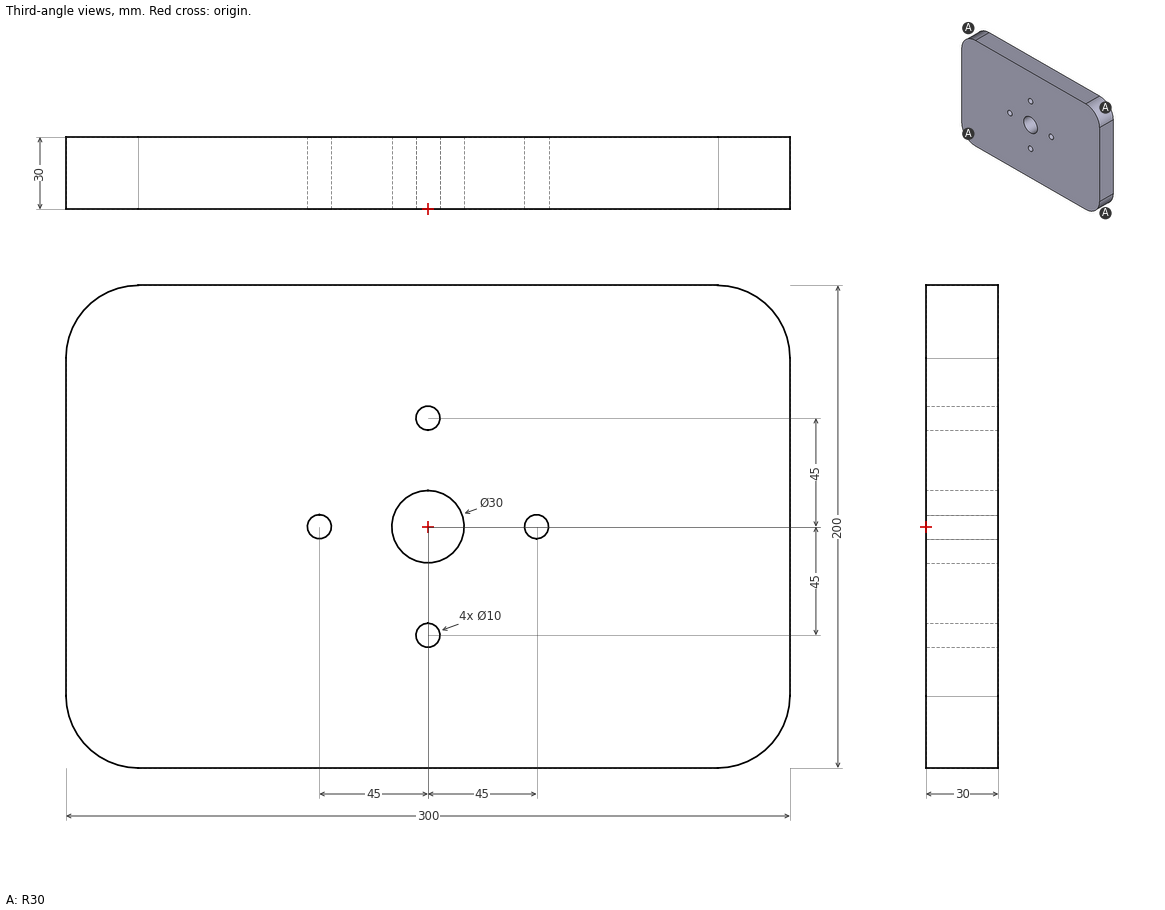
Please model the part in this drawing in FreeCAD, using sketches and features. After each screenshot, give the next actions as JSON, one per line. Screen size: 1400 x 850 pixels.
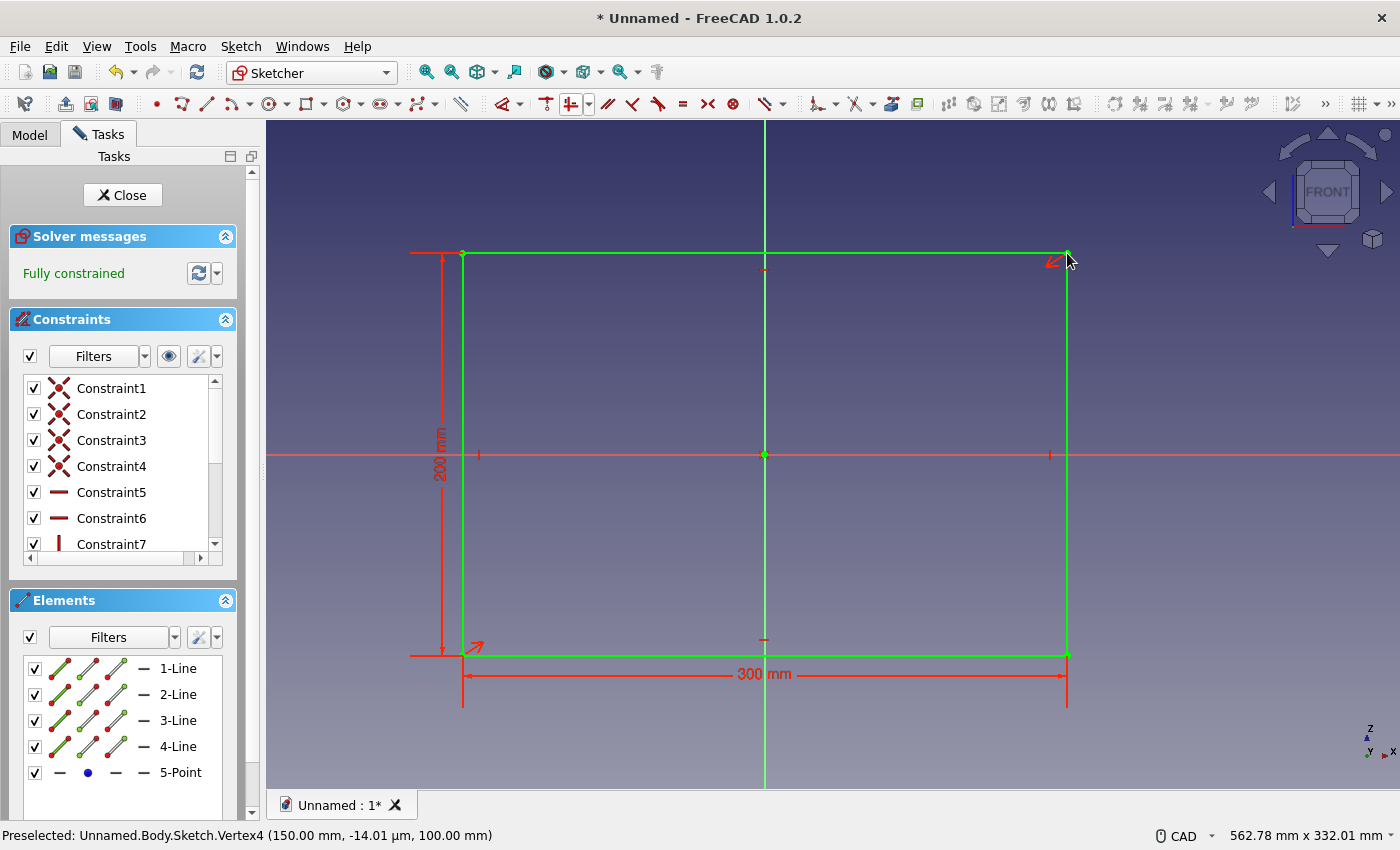
{"action": "left_click", "coordinate": [123, 195]}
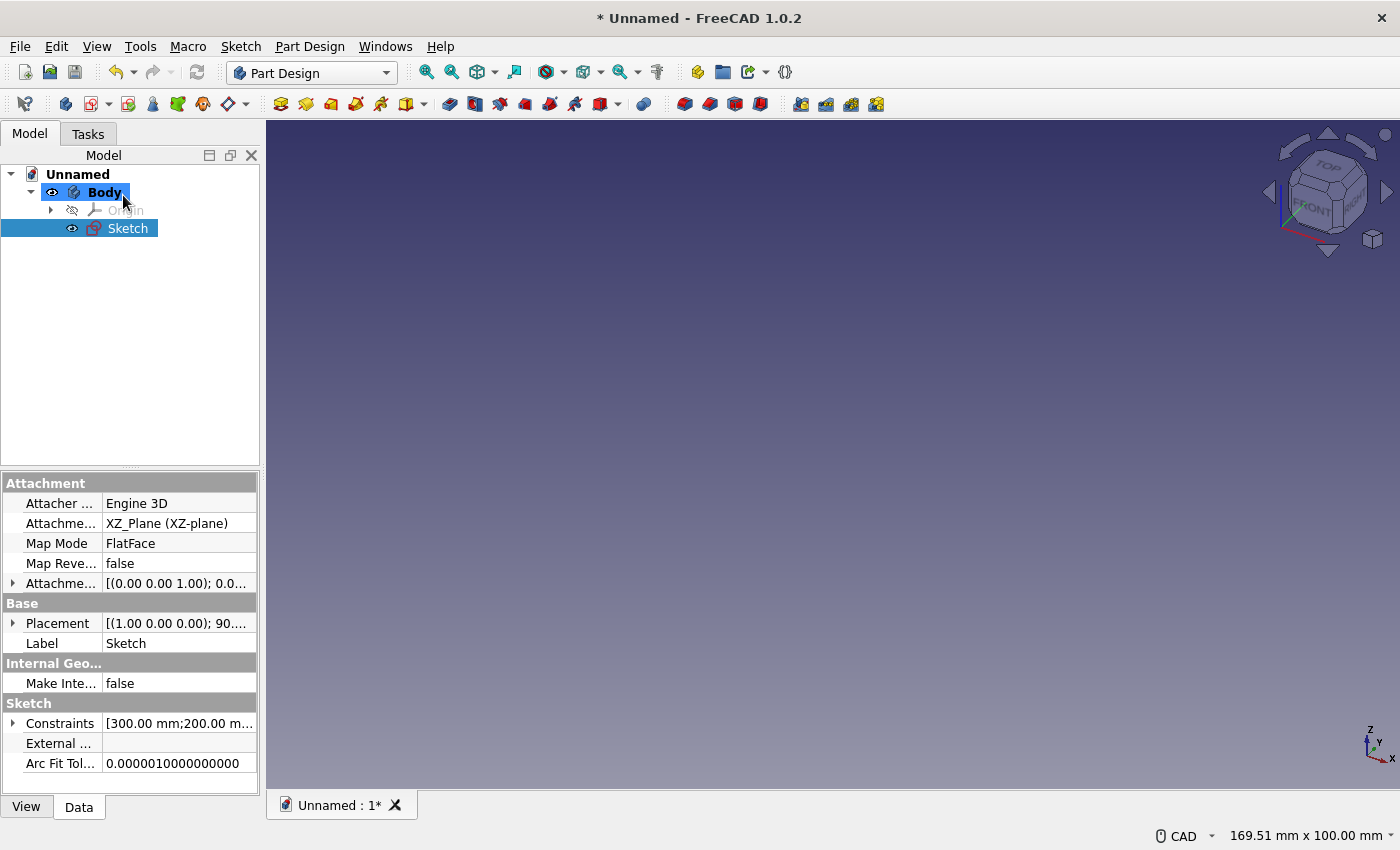
{"action": "left_click", "coordinate": [281, 104]}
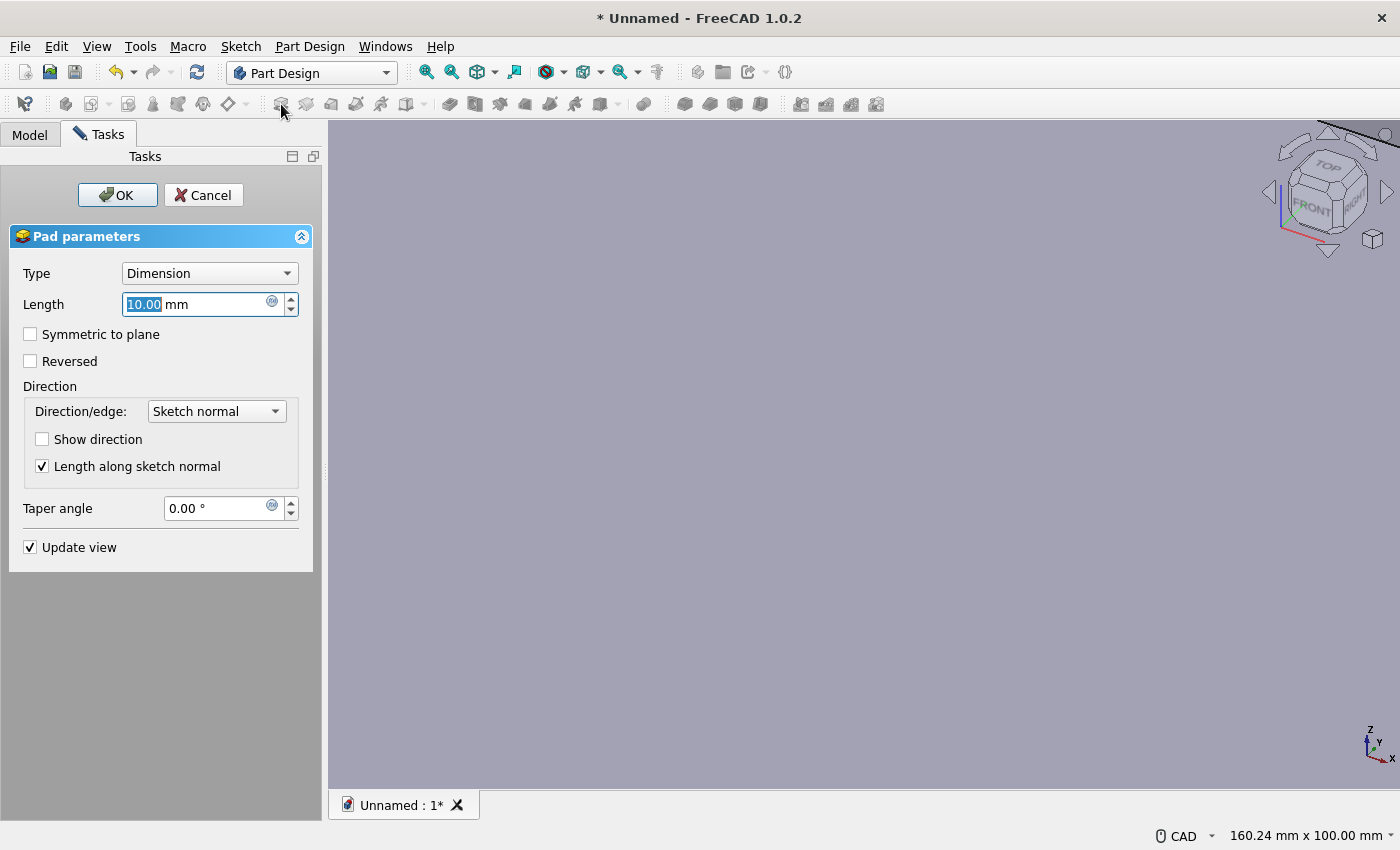
{"action": "type", "text": "30"}
{"action": "key", "text": "Tab"}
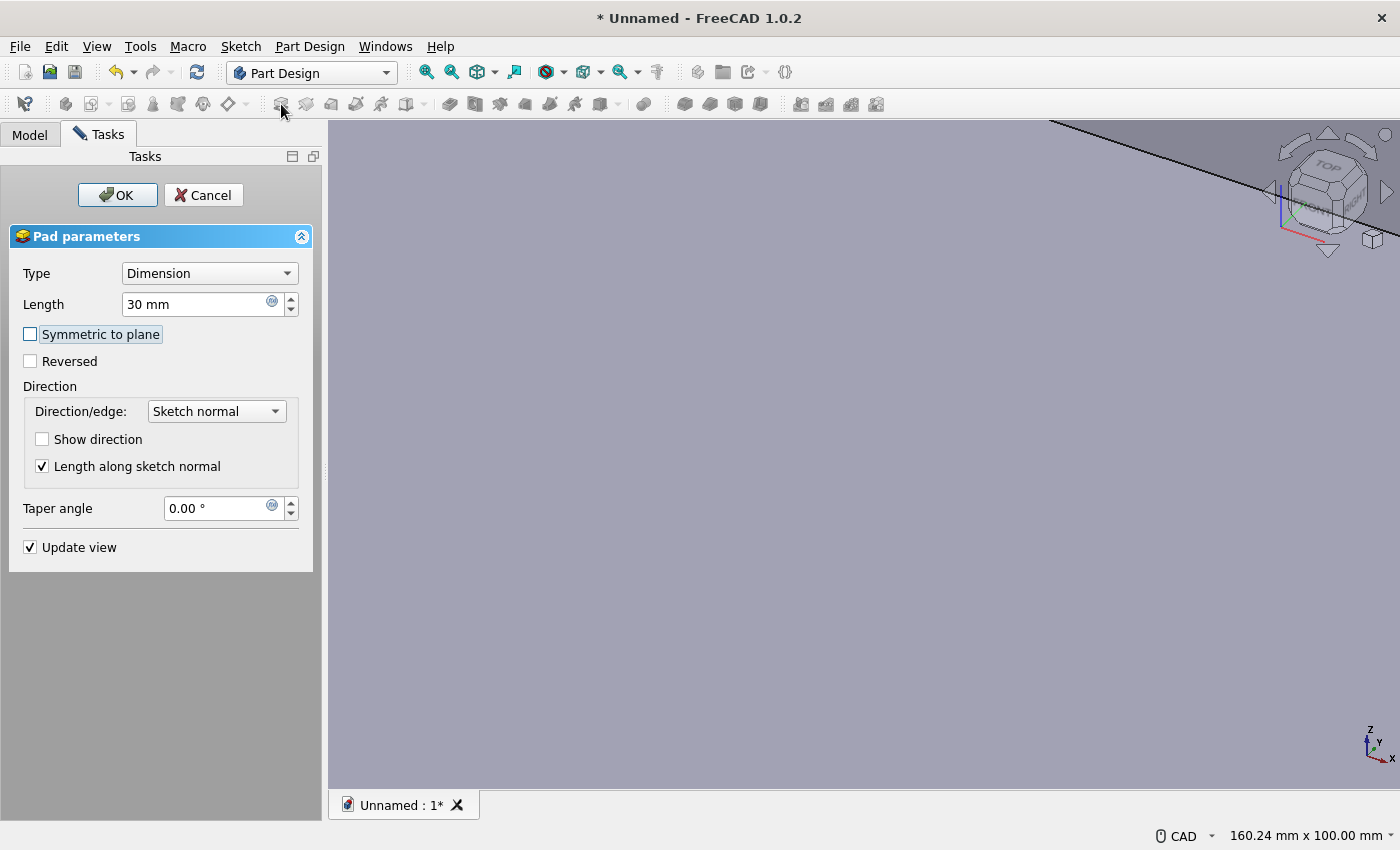
{"action": "left_click", "coordinate": [31, 361]}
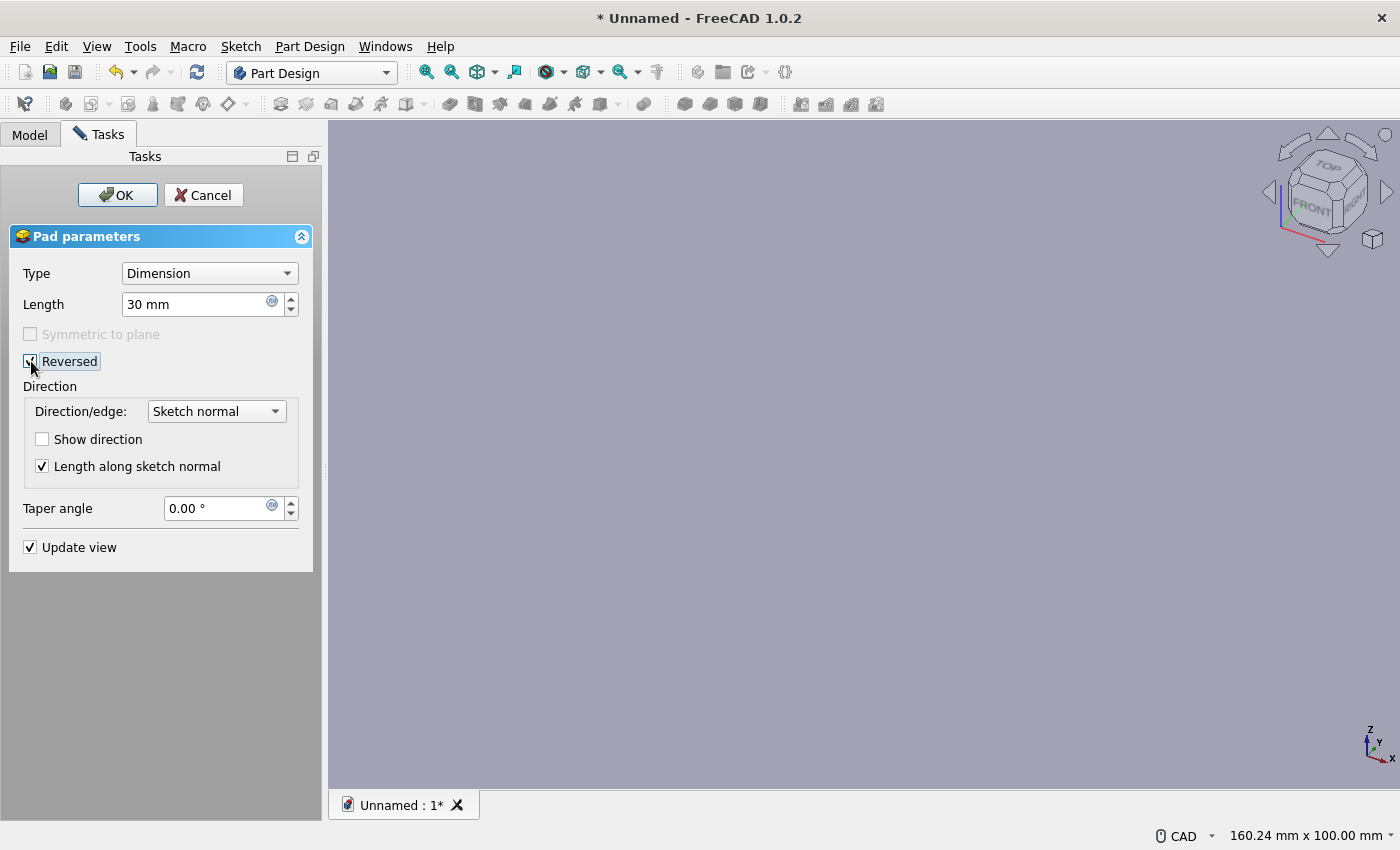
{"action": "left_click", "coordinate": [118, 195]}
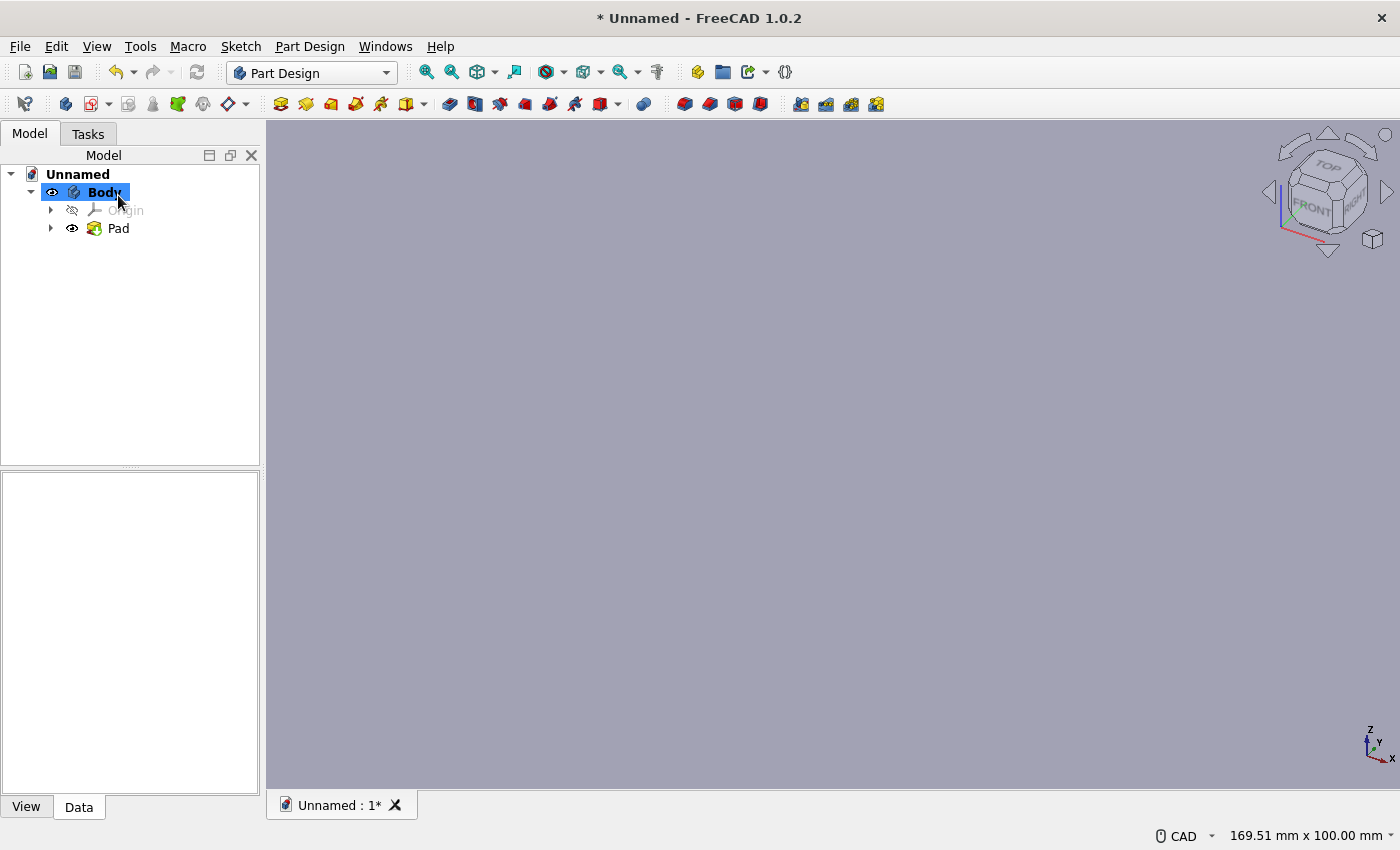
{"action": "key", "text": "v f"}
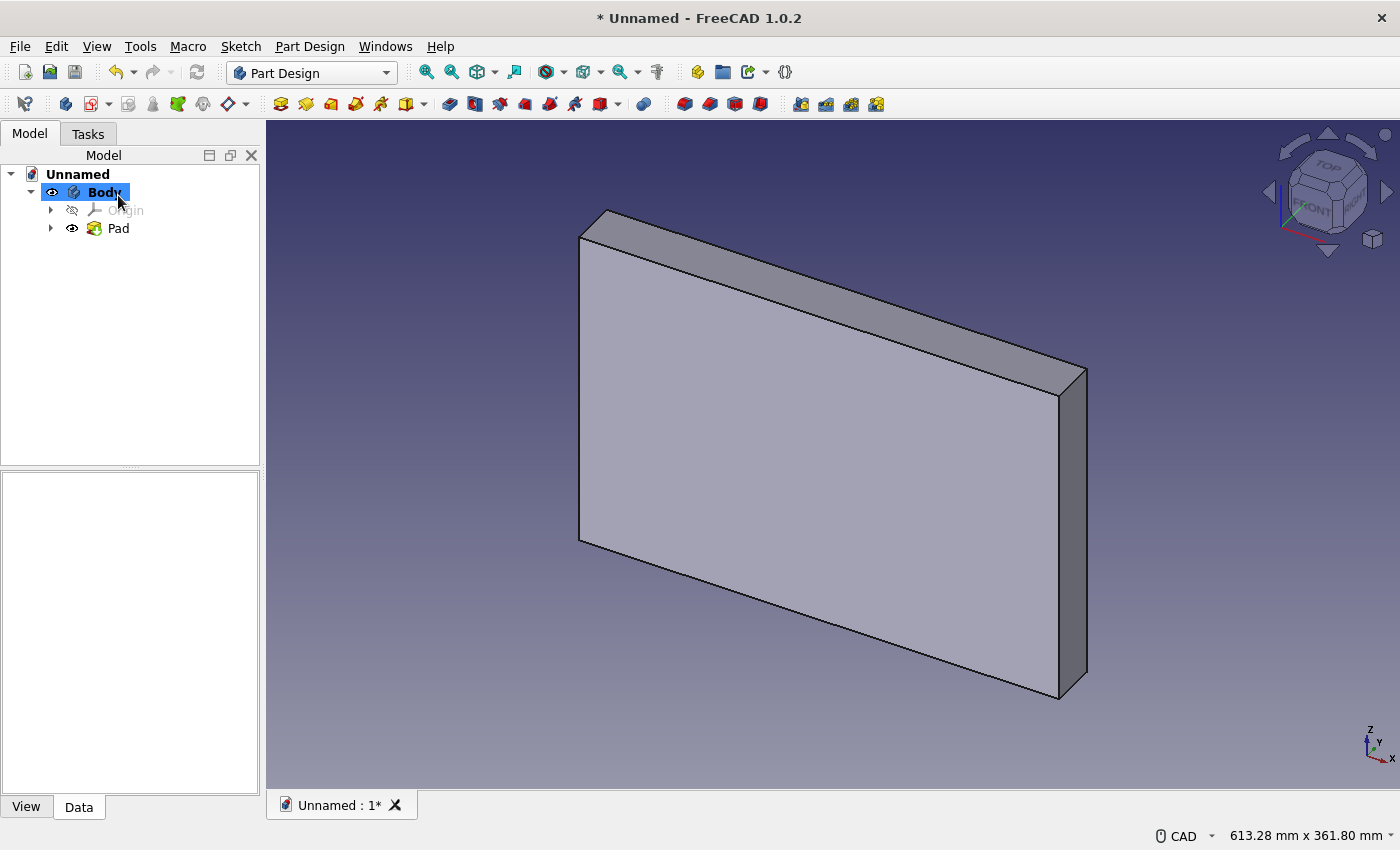
{"action": "key", "text": "4"}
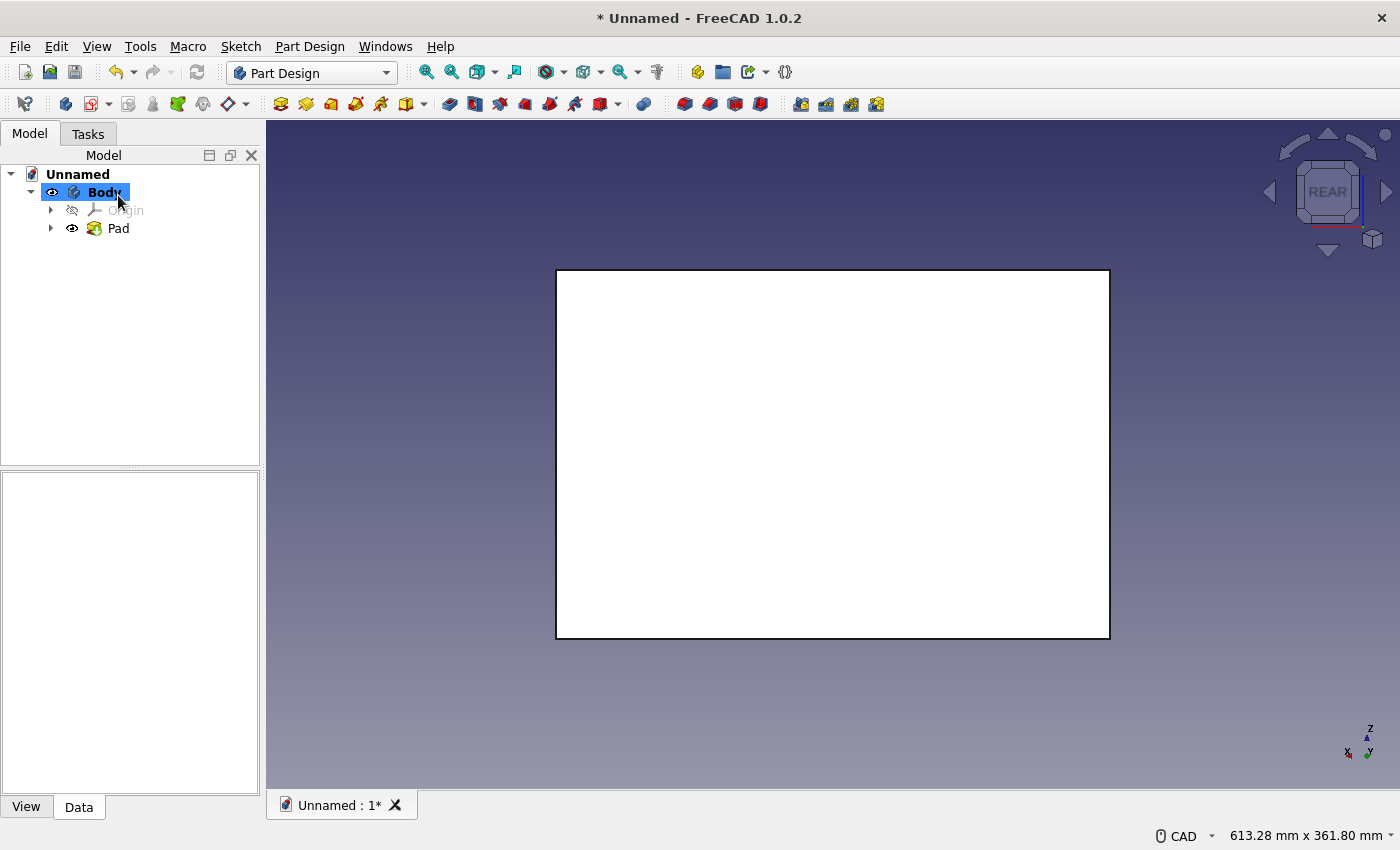
{"action": "left_click", "coordinate": [754, 453]}